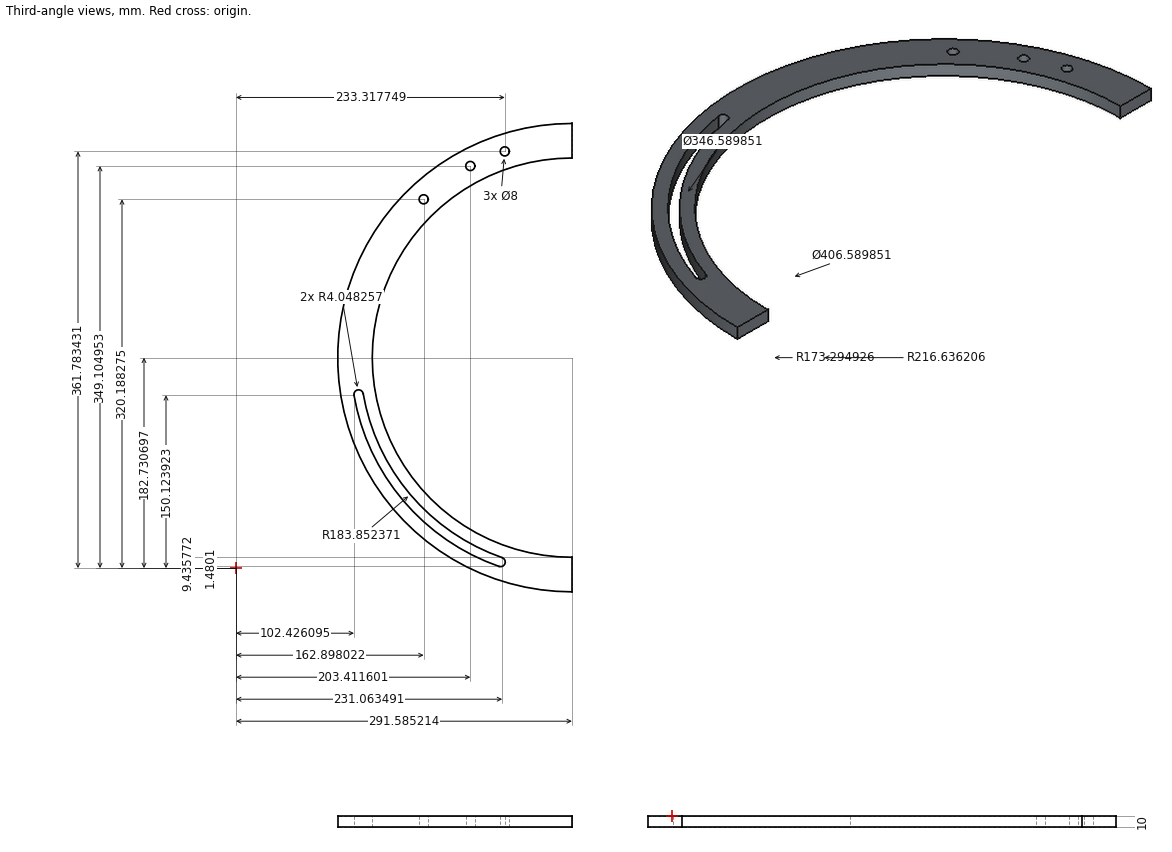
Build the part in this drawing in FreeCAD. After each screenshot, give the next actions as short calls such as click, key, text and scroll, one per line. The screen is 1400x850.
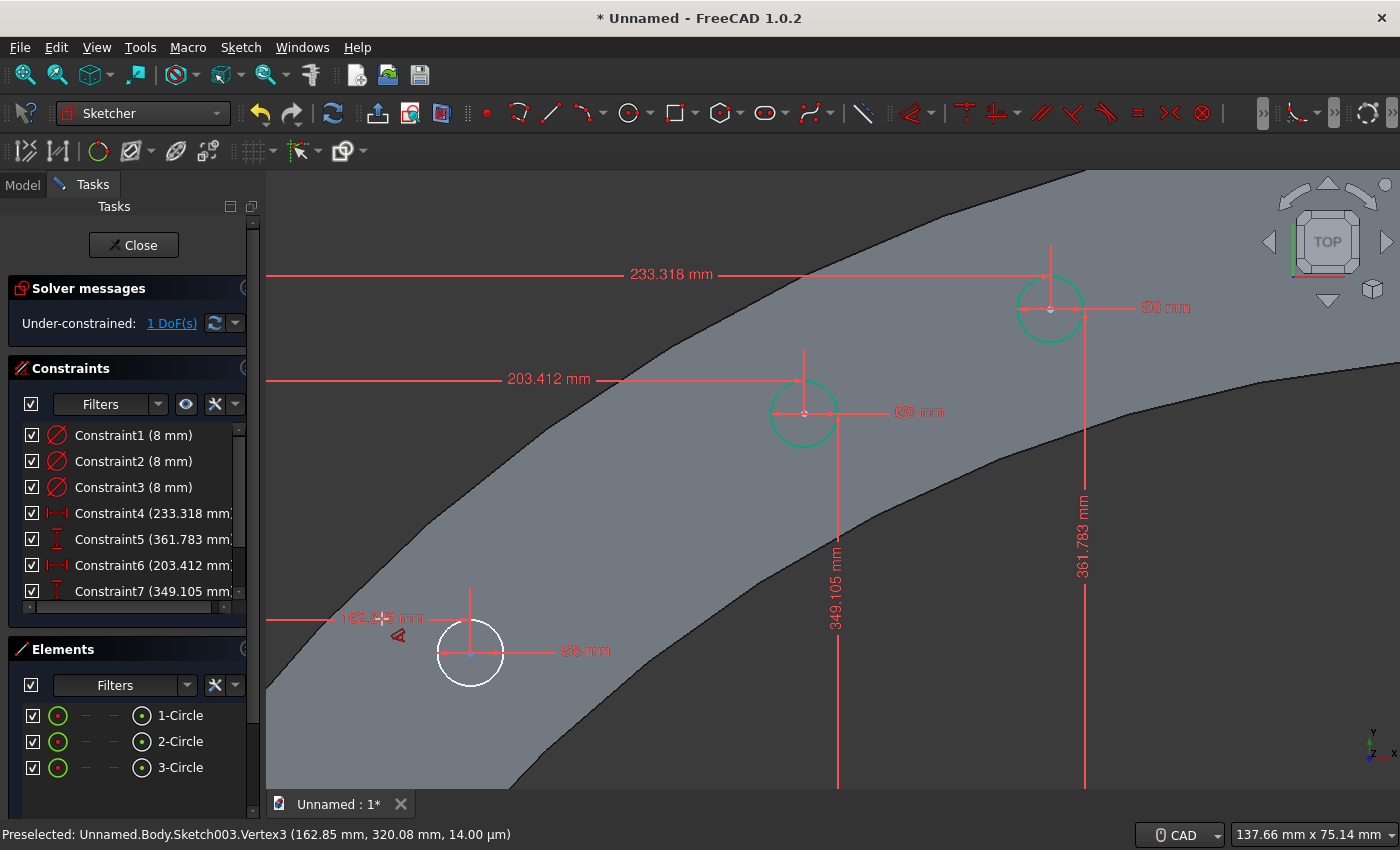
click(470, 653)
click(504, 707)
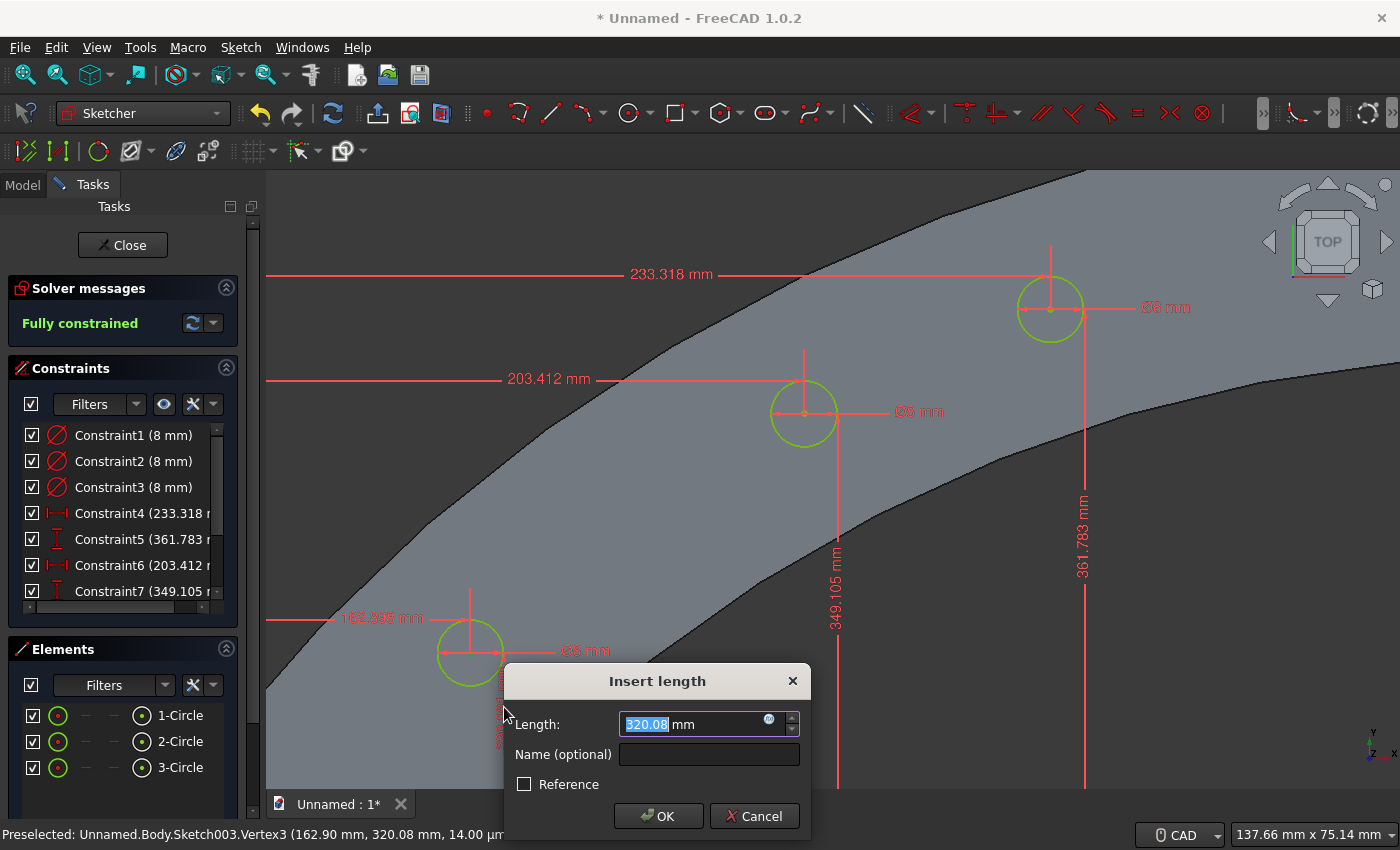
text(320.188275)
key(Return)
key(Escape)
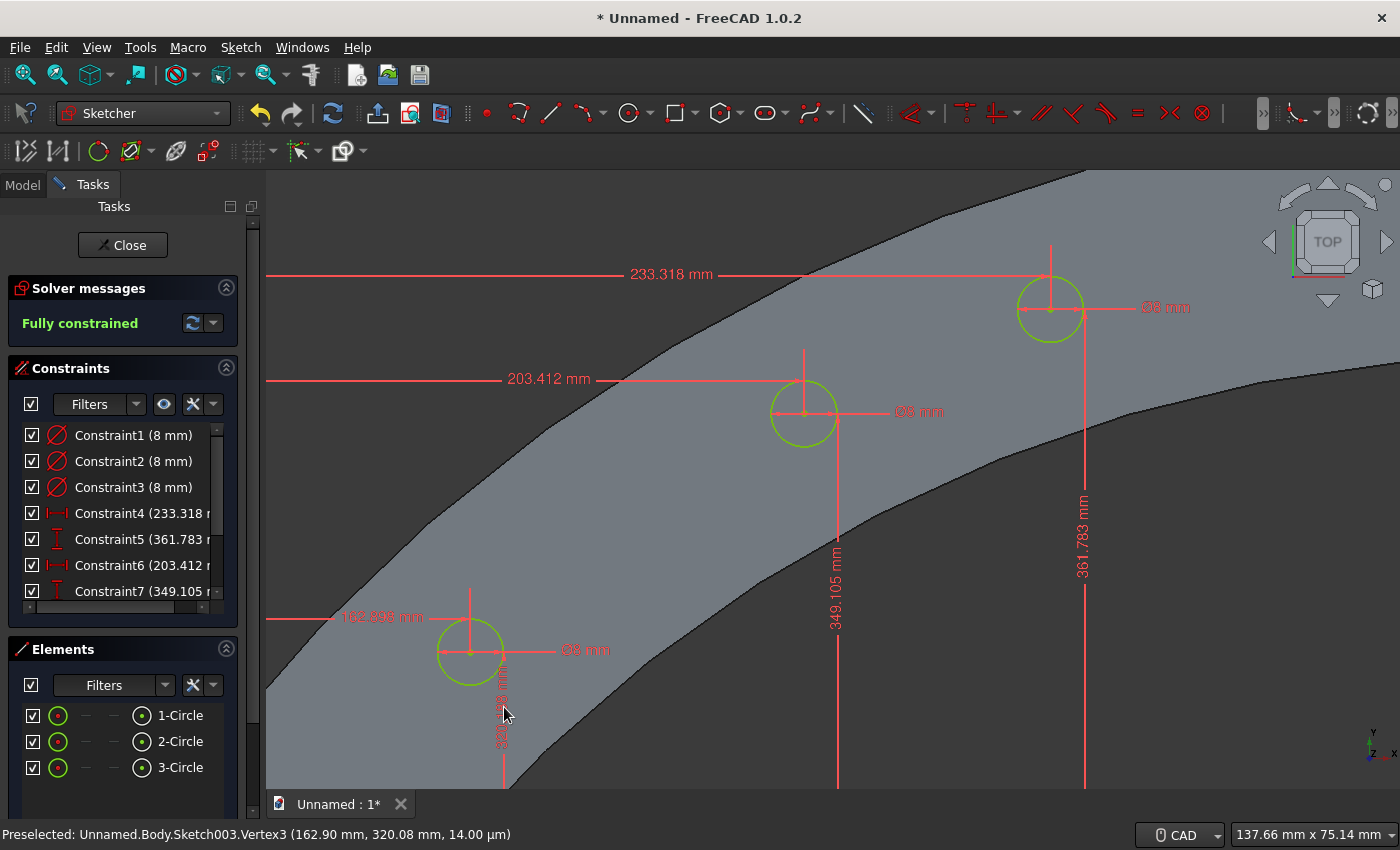
click(123, 245)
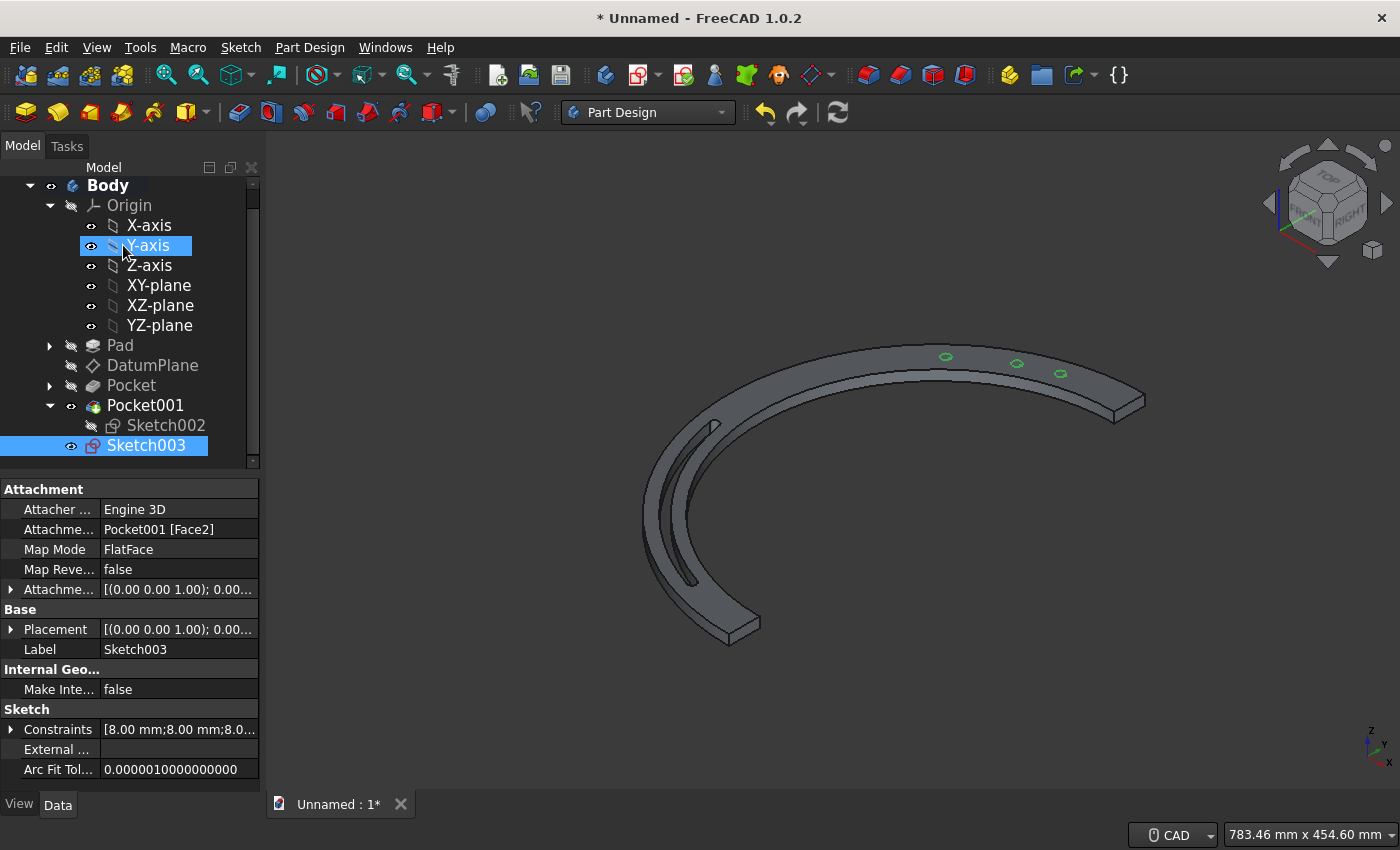
click(240, 112)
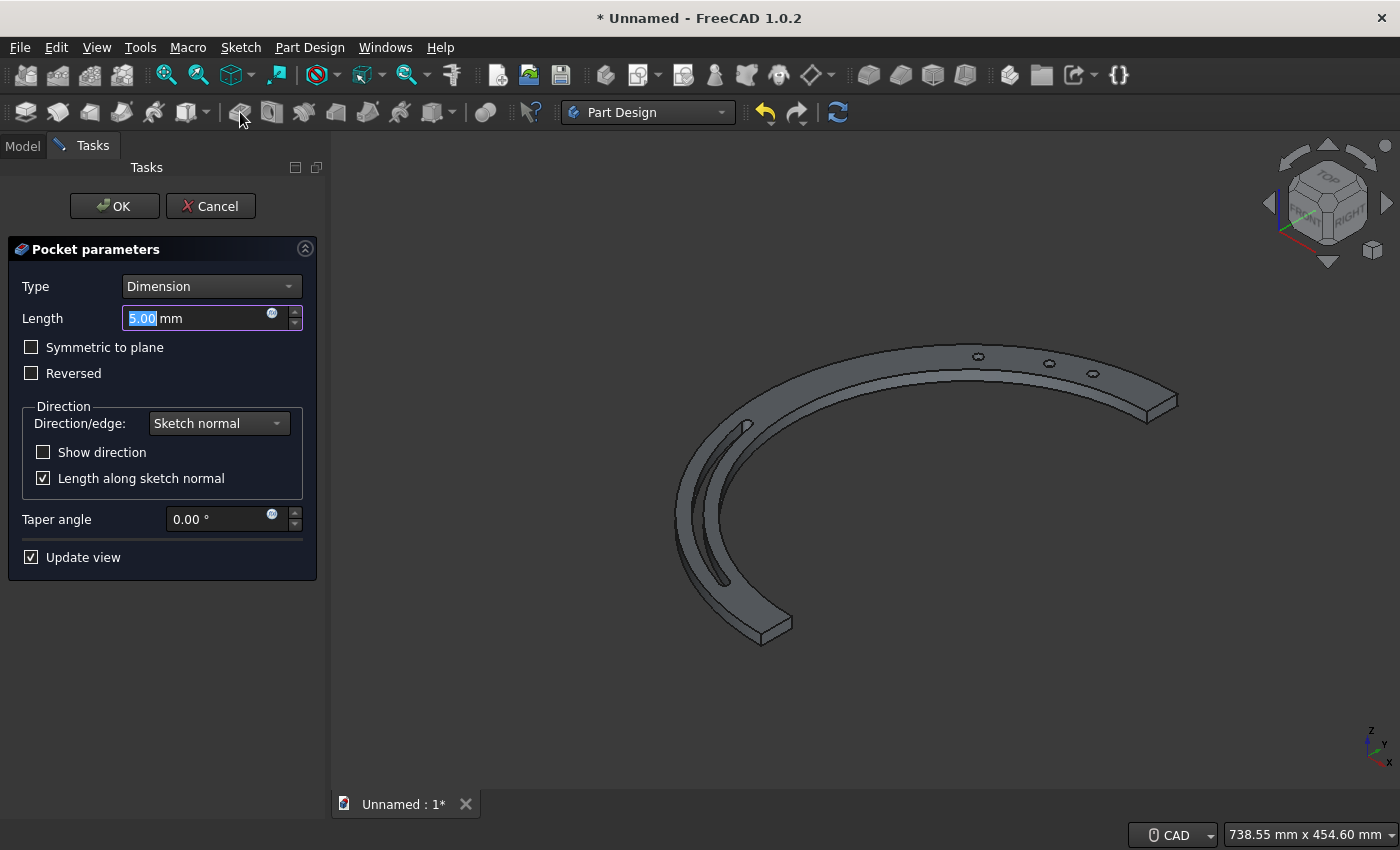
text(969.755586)
key(Tab)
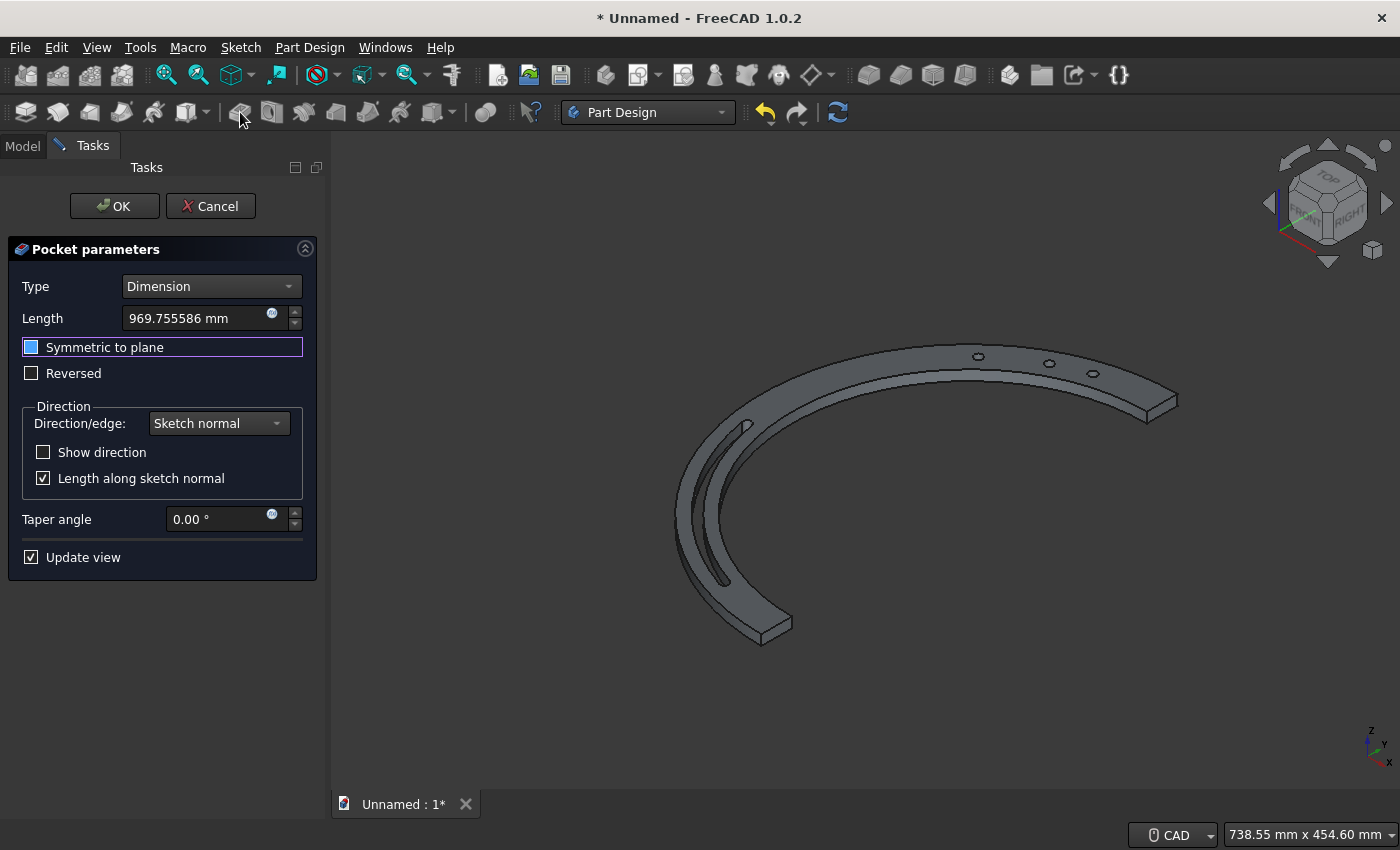
click(30, 347)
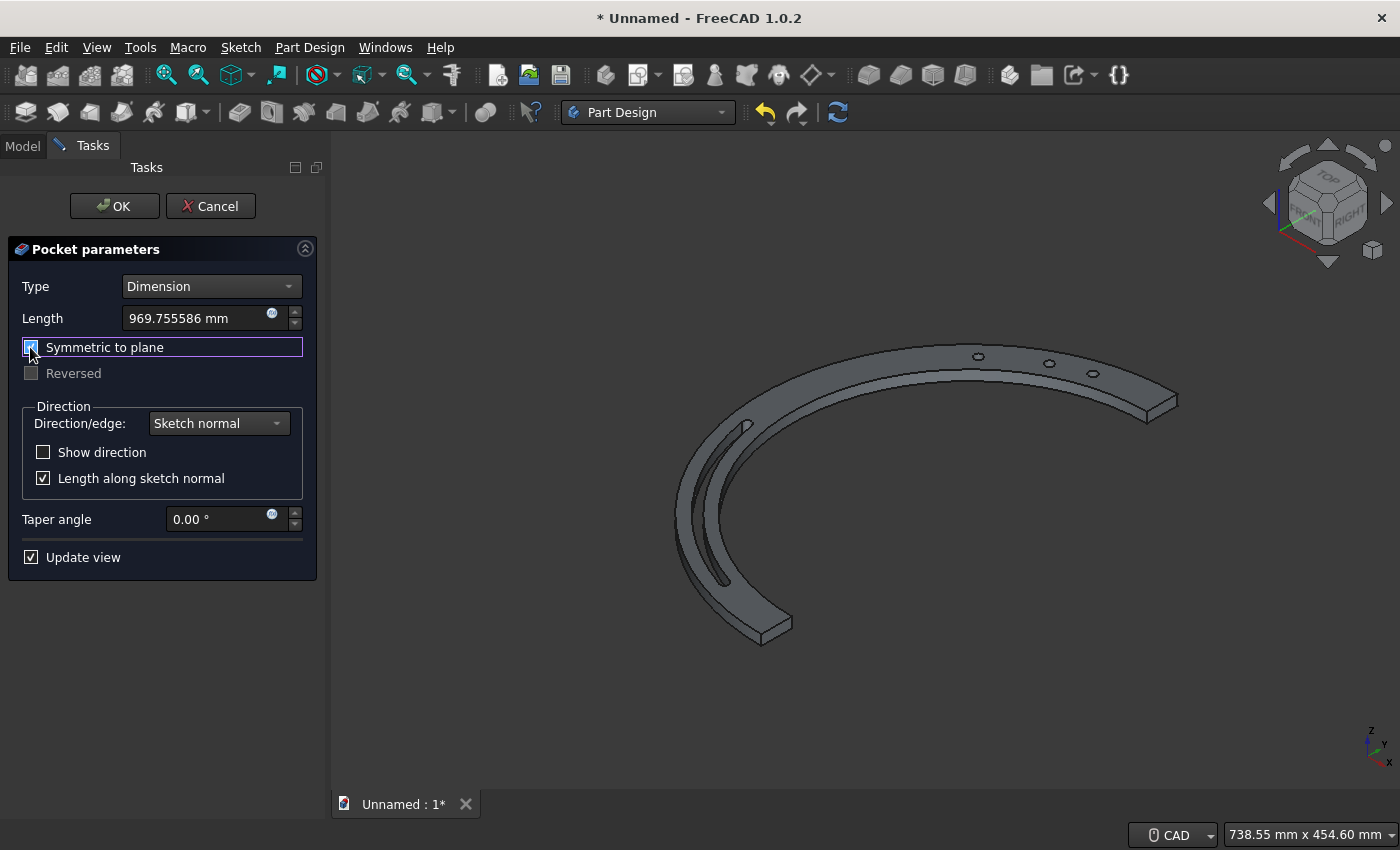
click(115, 206)